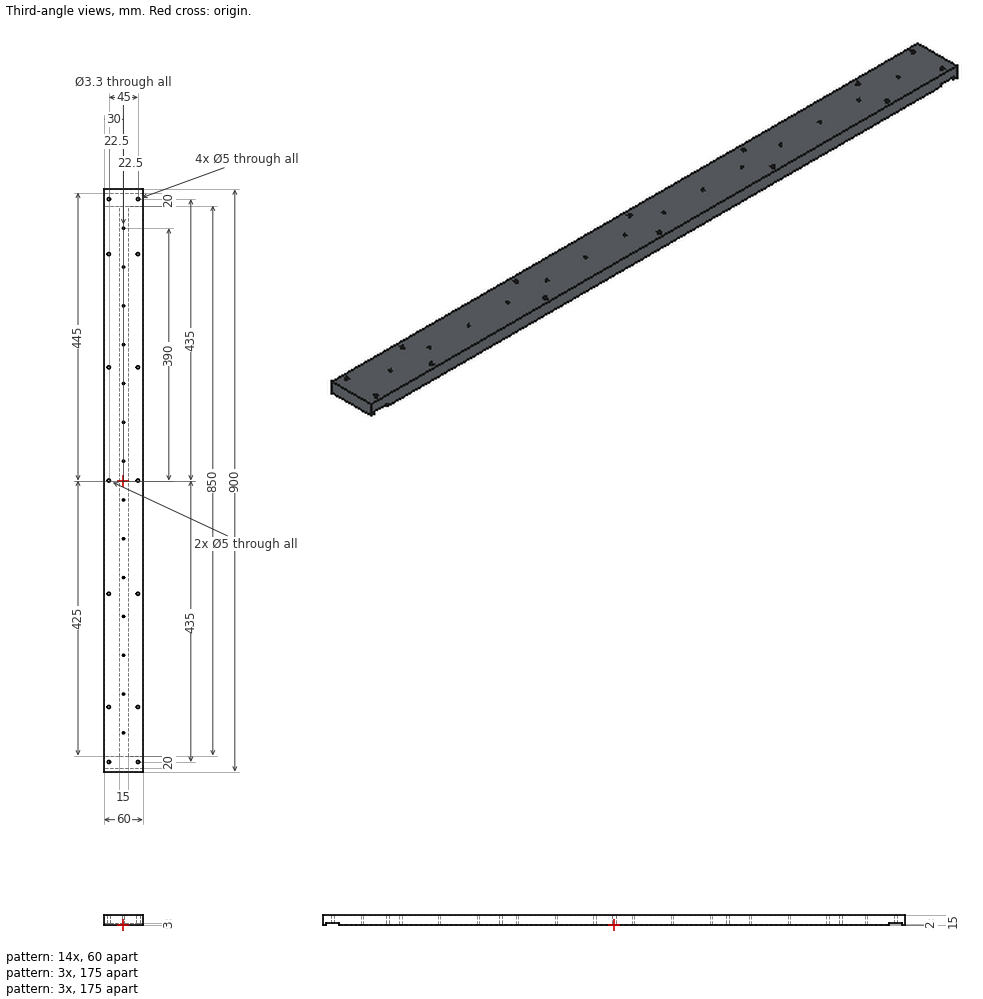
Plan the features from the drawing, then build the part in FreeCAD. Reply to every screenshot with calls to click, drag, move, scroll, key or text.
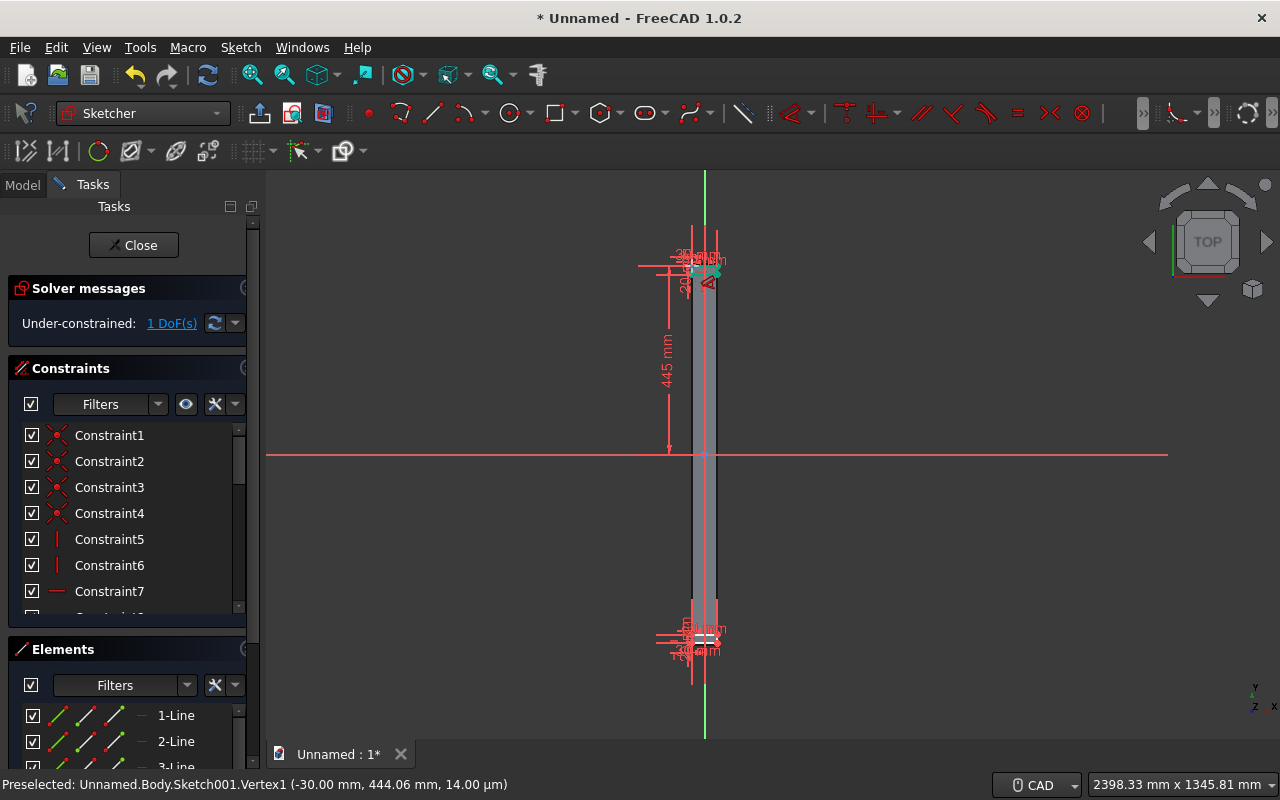
scroll(692, 635, up, 2)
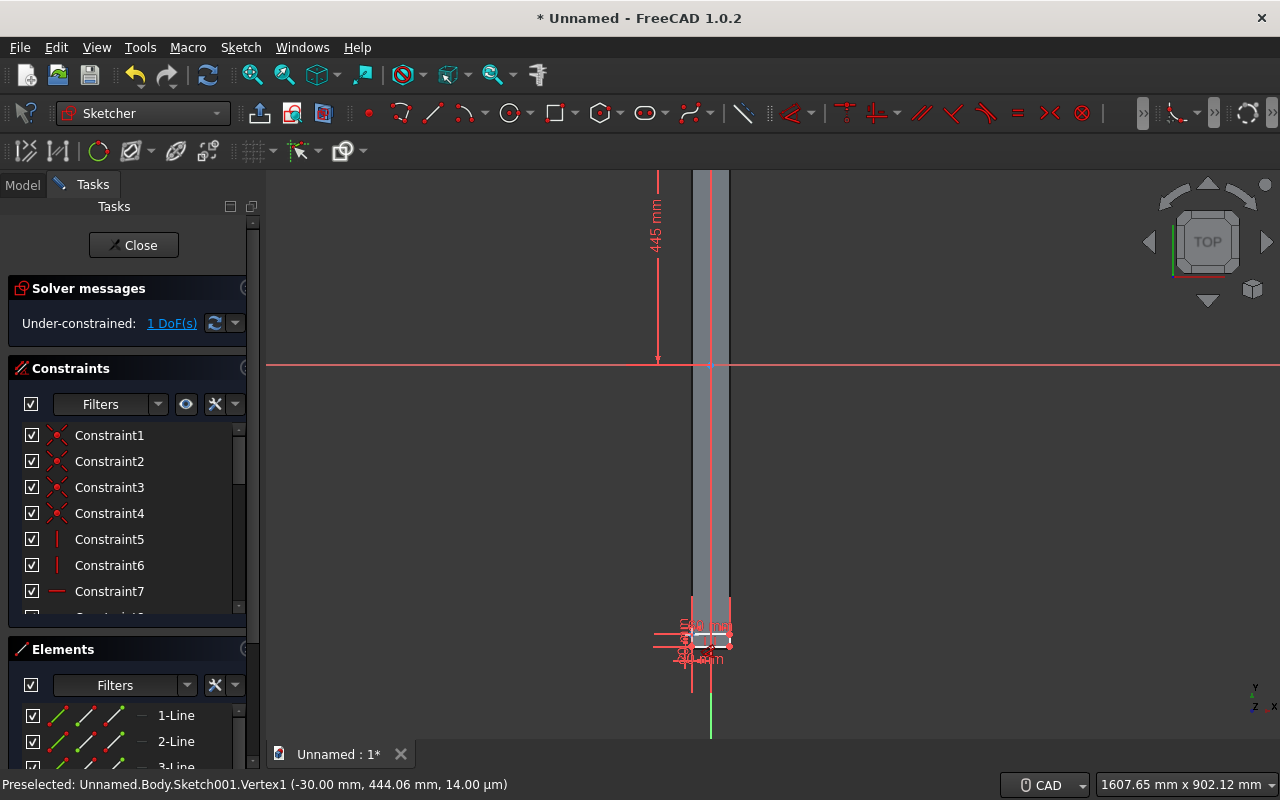
click(692, 634)
click(658, 500)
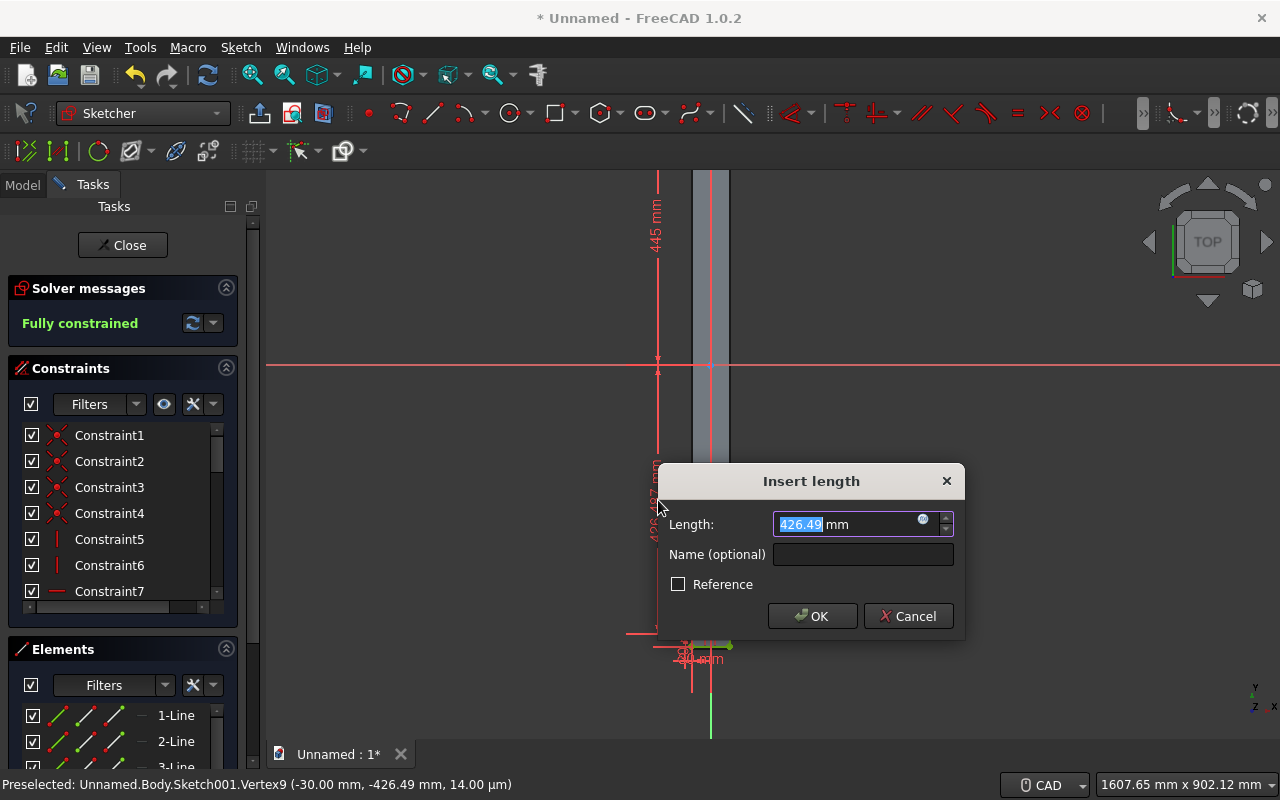
text(425)
key(Return)
key(Escape)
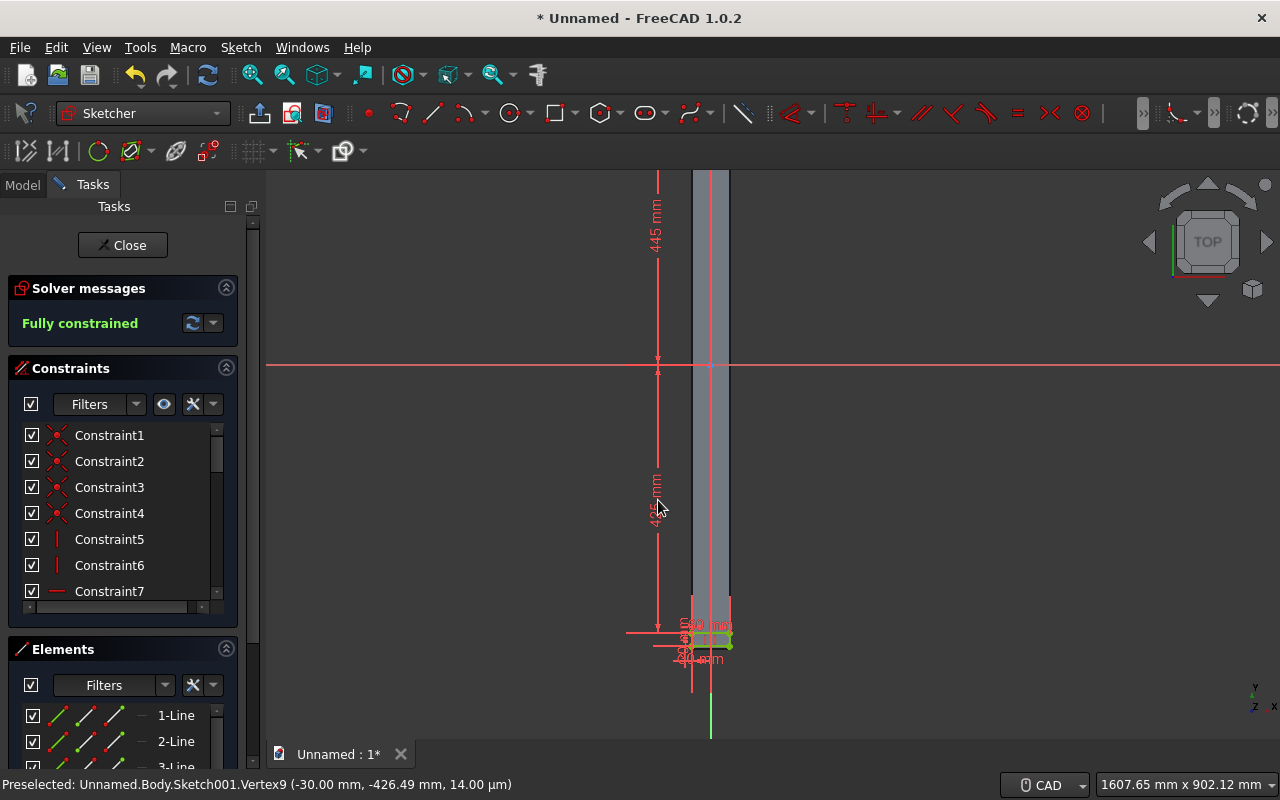
click(123, 245)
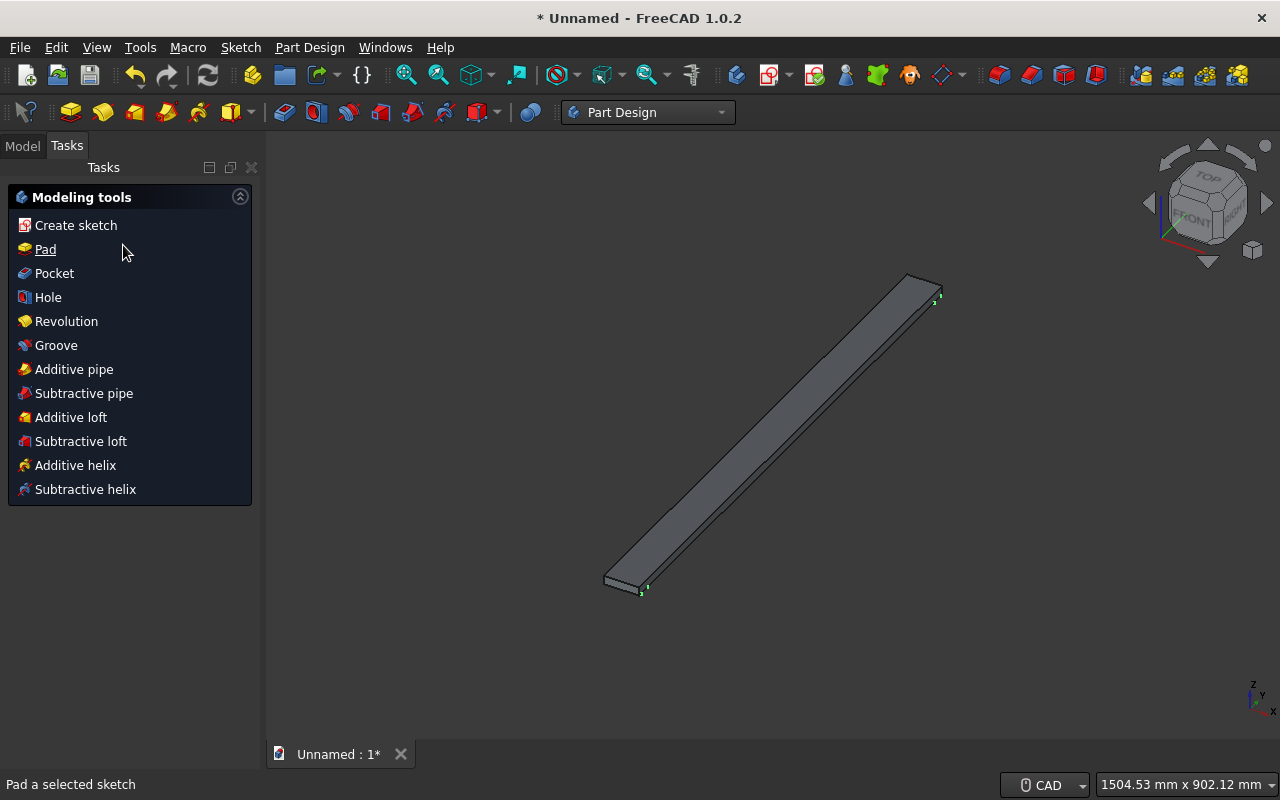
click(286, 112)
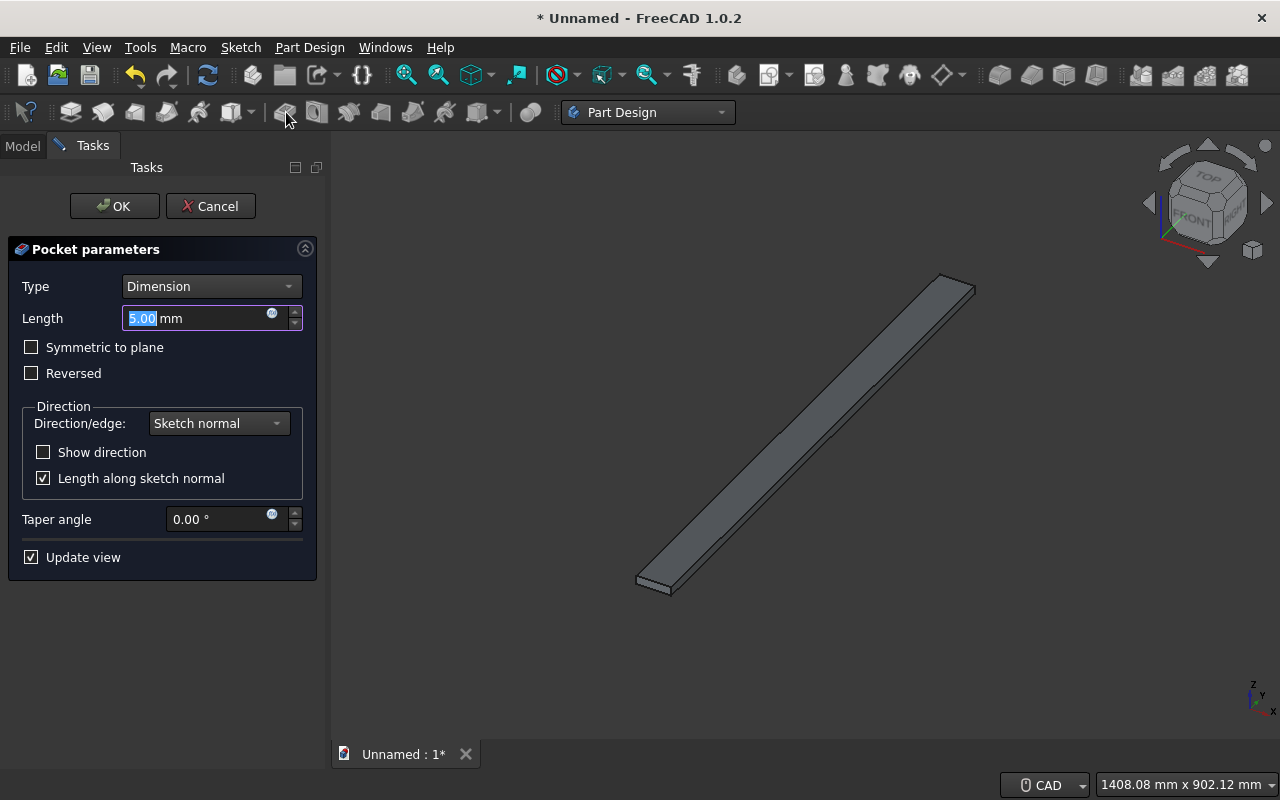
text(3)
key(Tab)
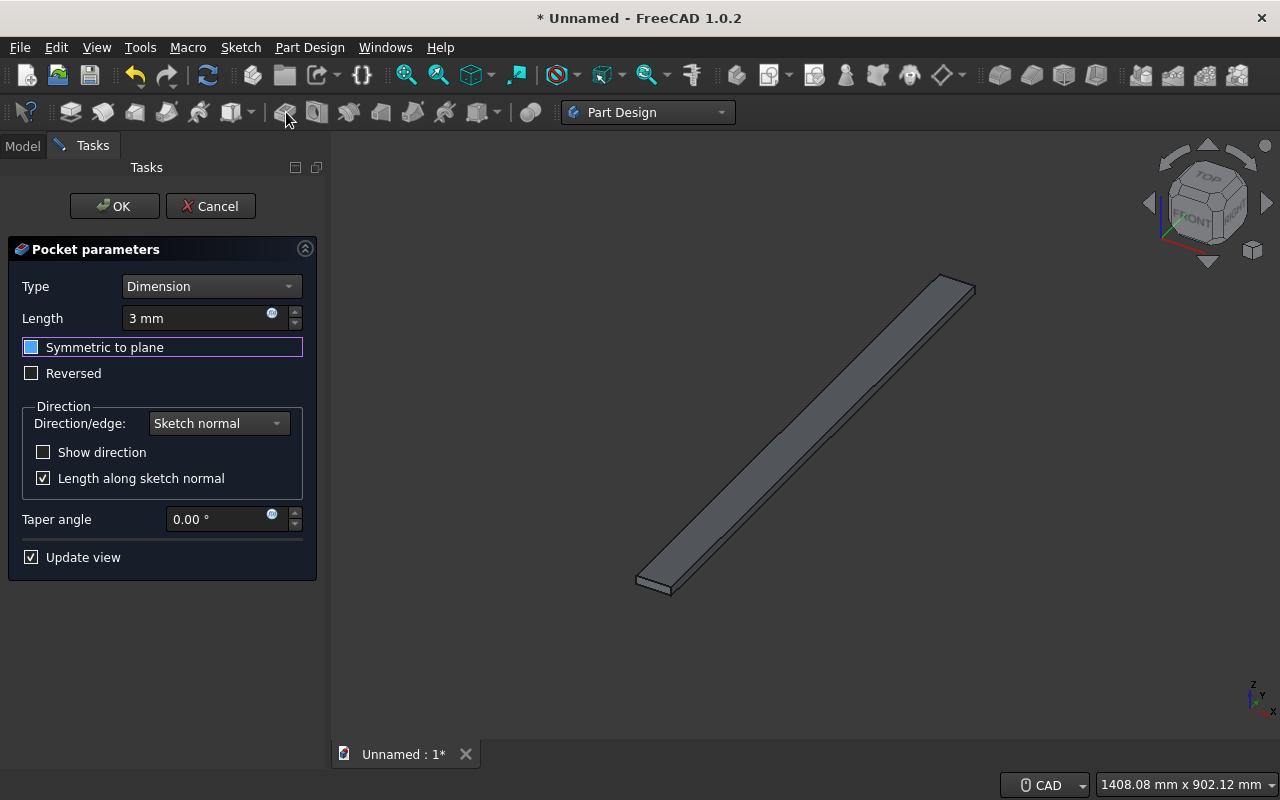
click(30, 373)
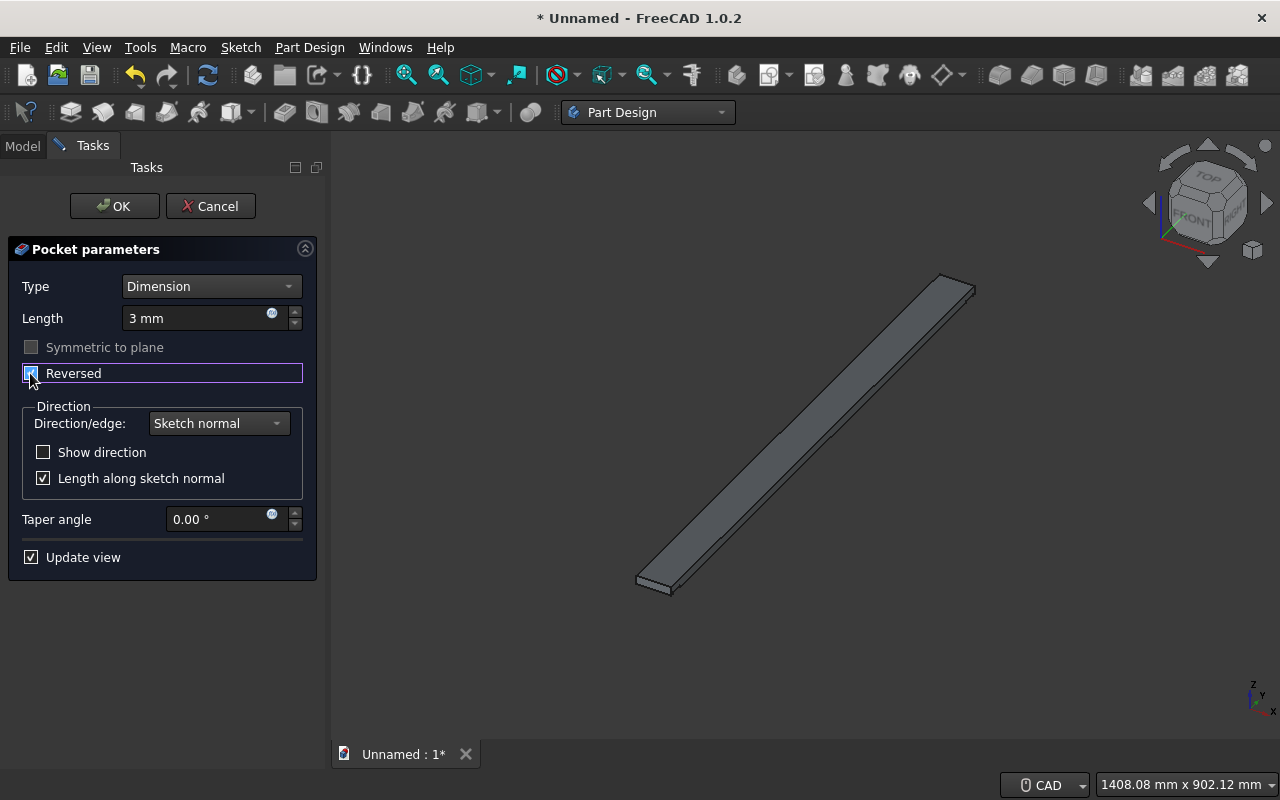
click(115, 206)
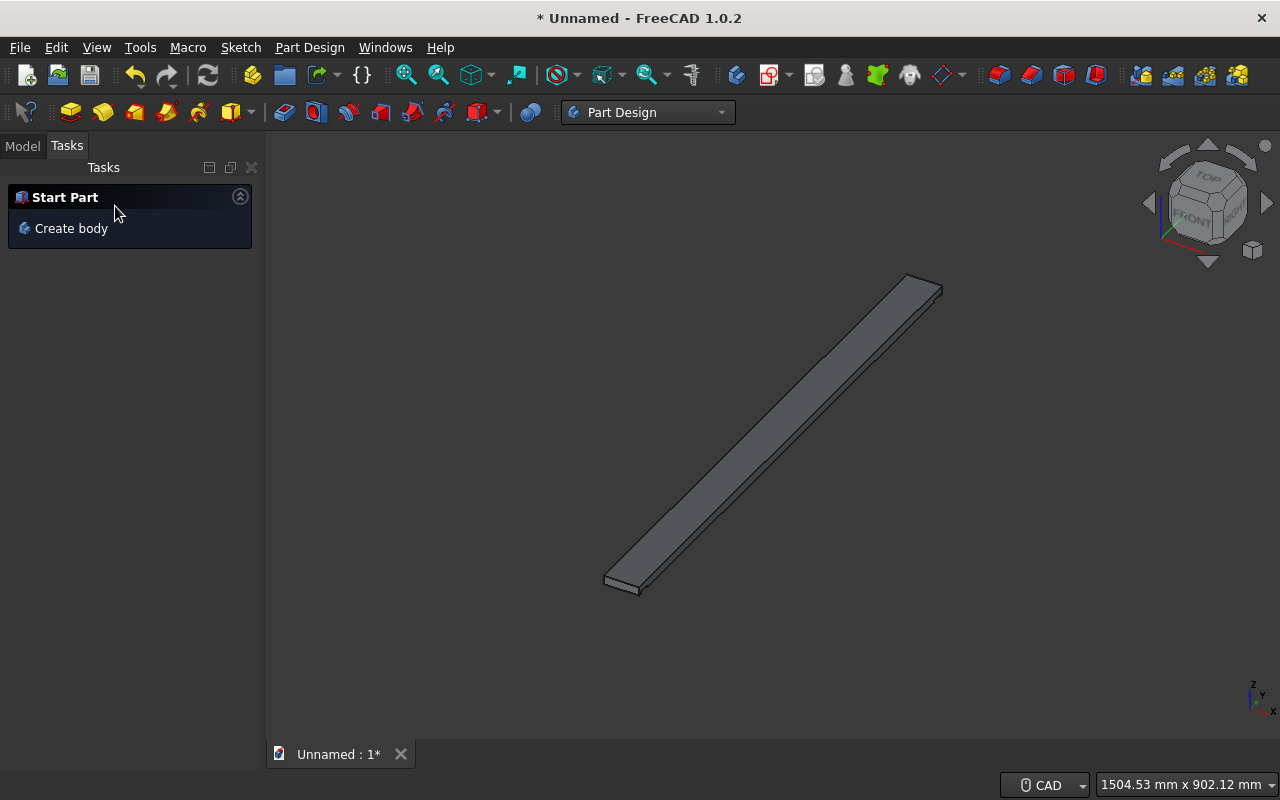
click(770, 76)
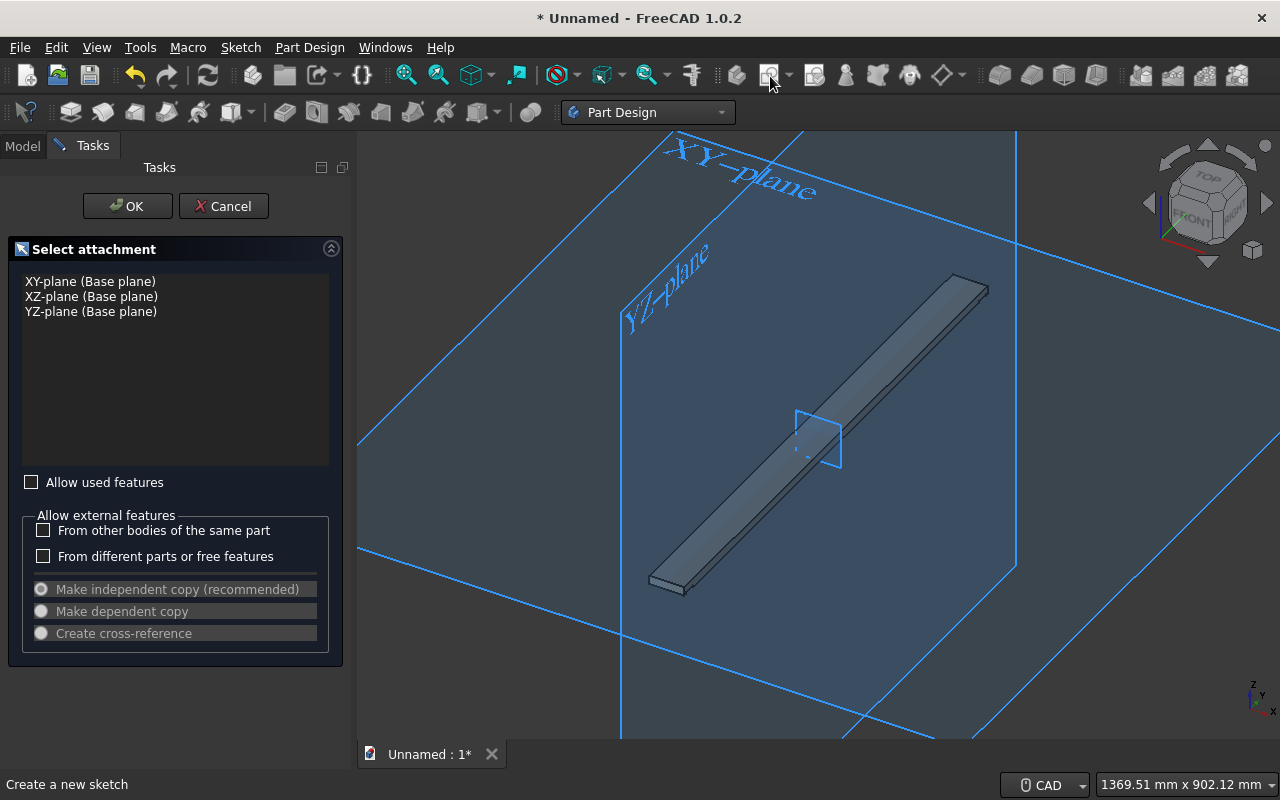
click(82, 282)